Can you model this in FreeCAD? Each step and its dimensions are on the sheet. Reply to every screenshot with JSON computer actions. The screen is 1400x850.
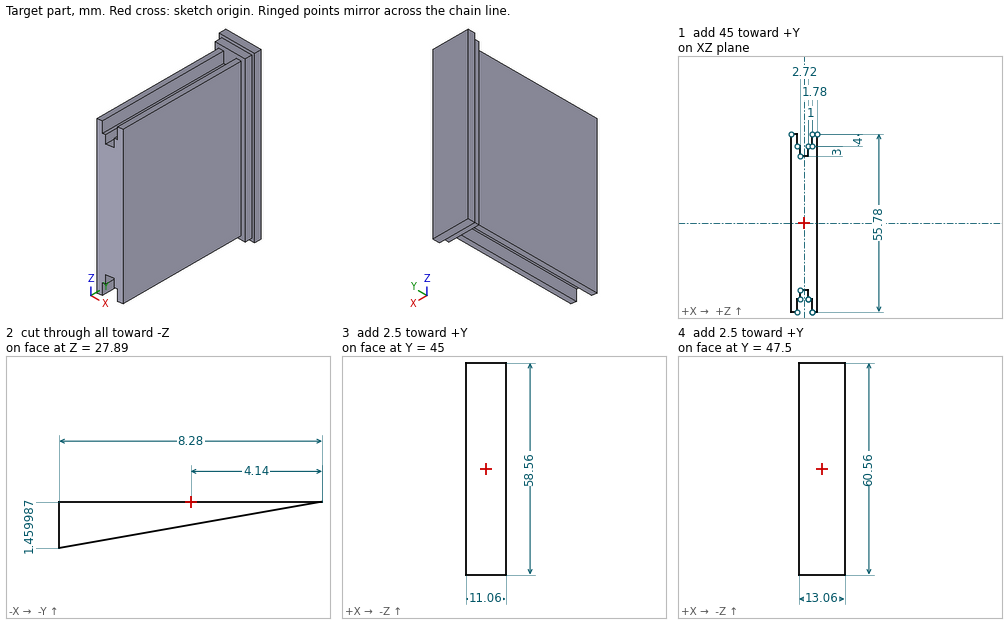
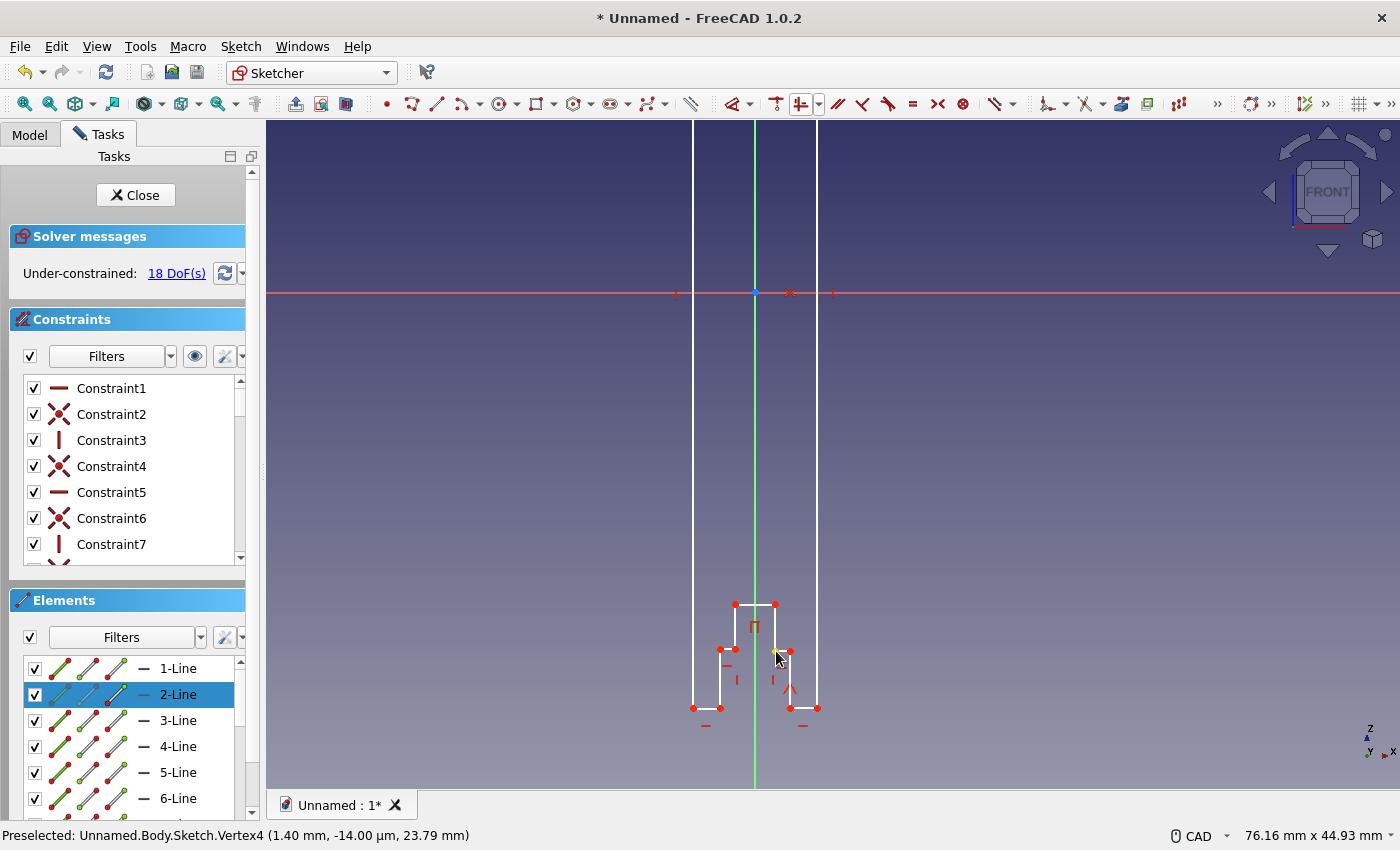
{"action": "left_click", "coordinate": [775, 651]}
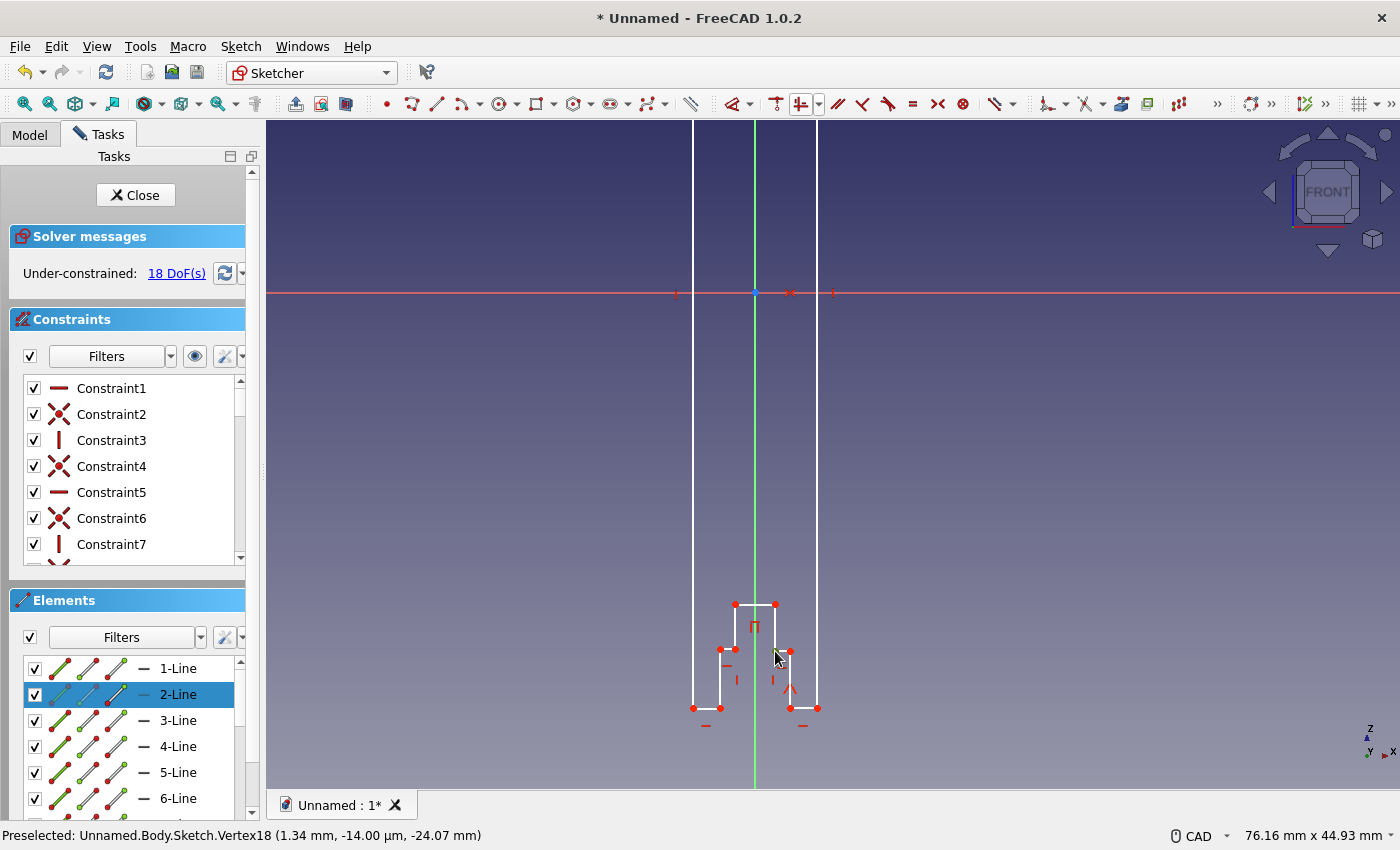
{"action": "left_click", "coordinate": [361, 293]}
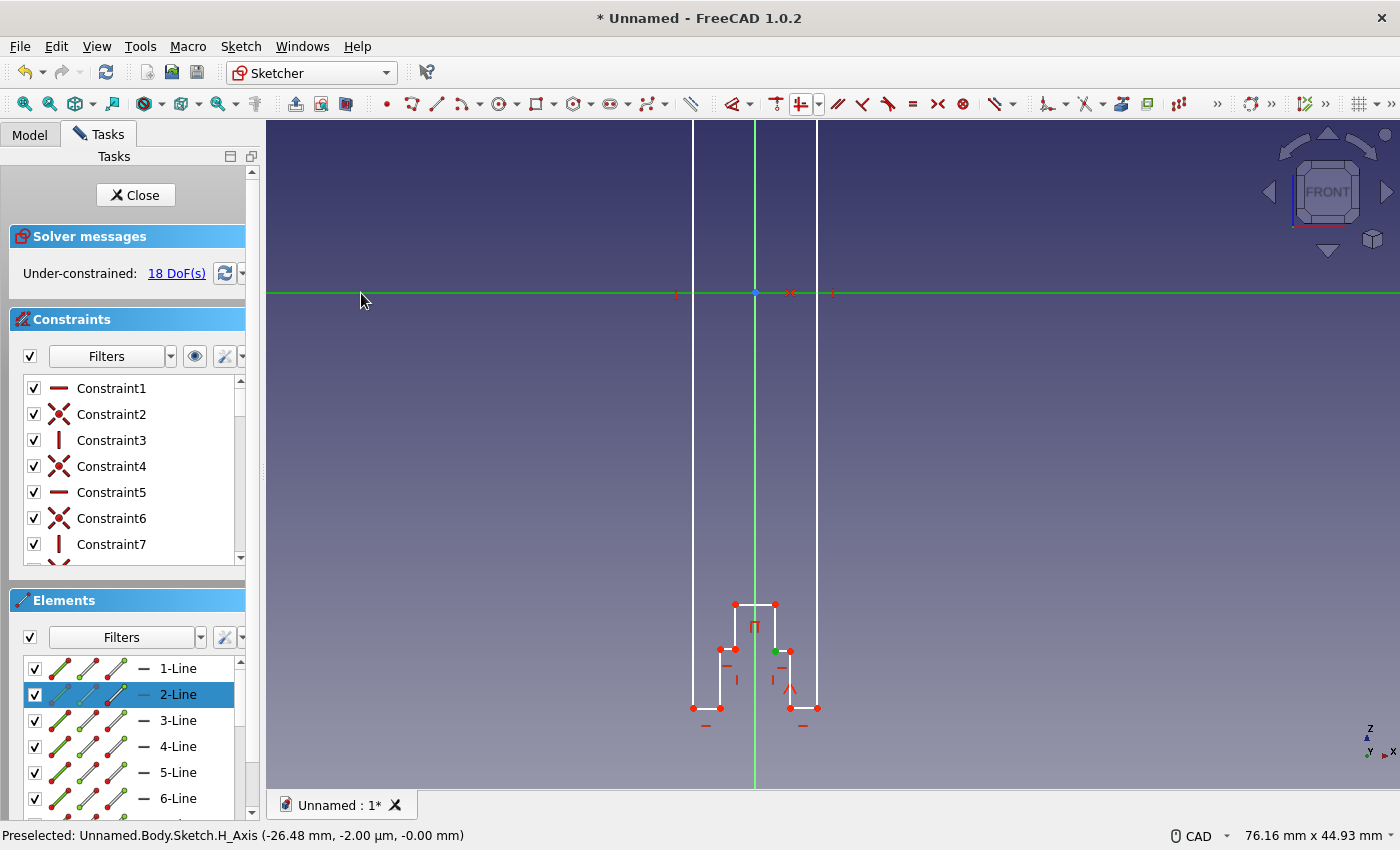
{"action": "left_click", "coordinate": [938, 104]}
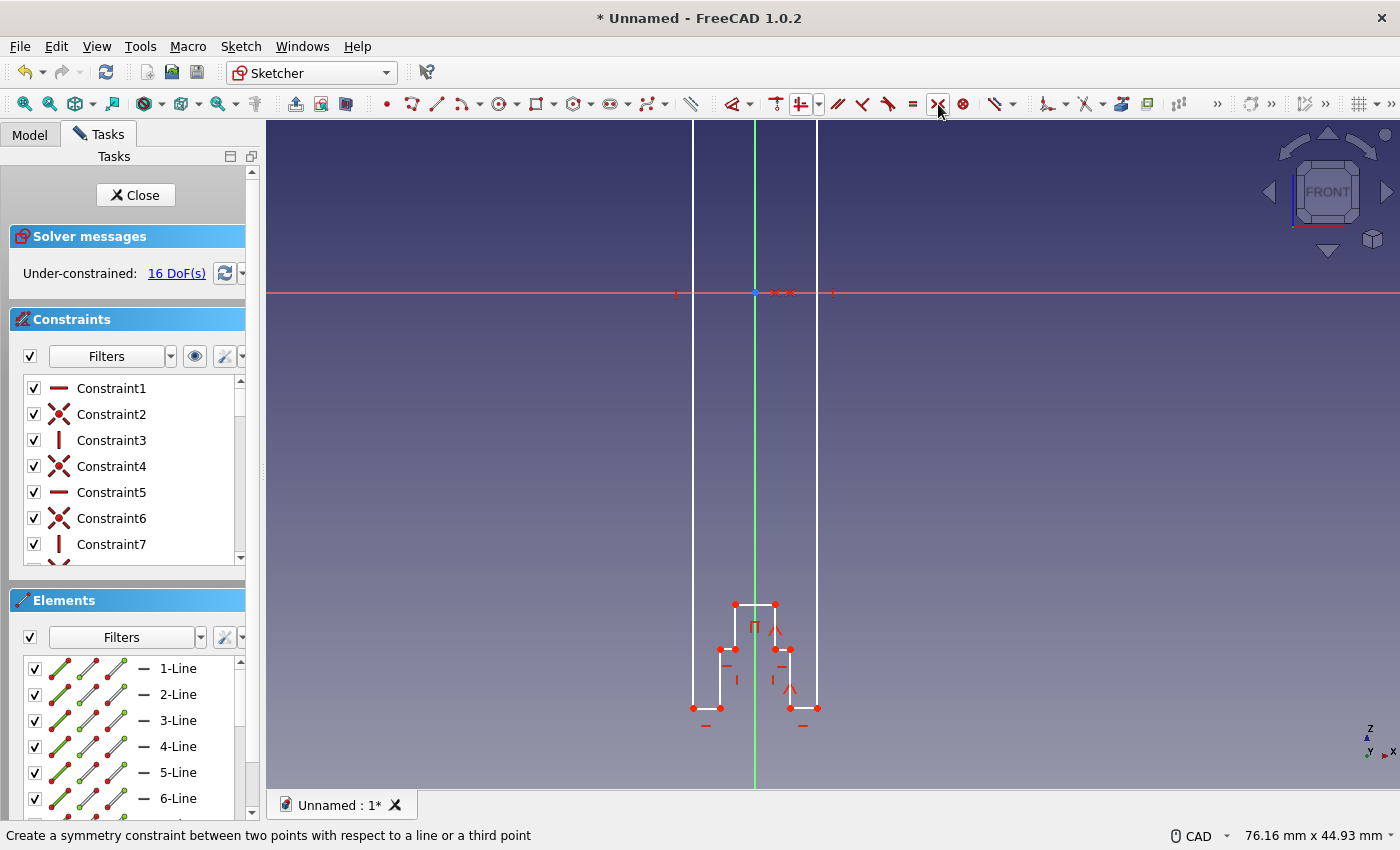
{"action": "scroll", "coordinate": [776, 651], "scroll_direction": "down", "scroll_amount": 3}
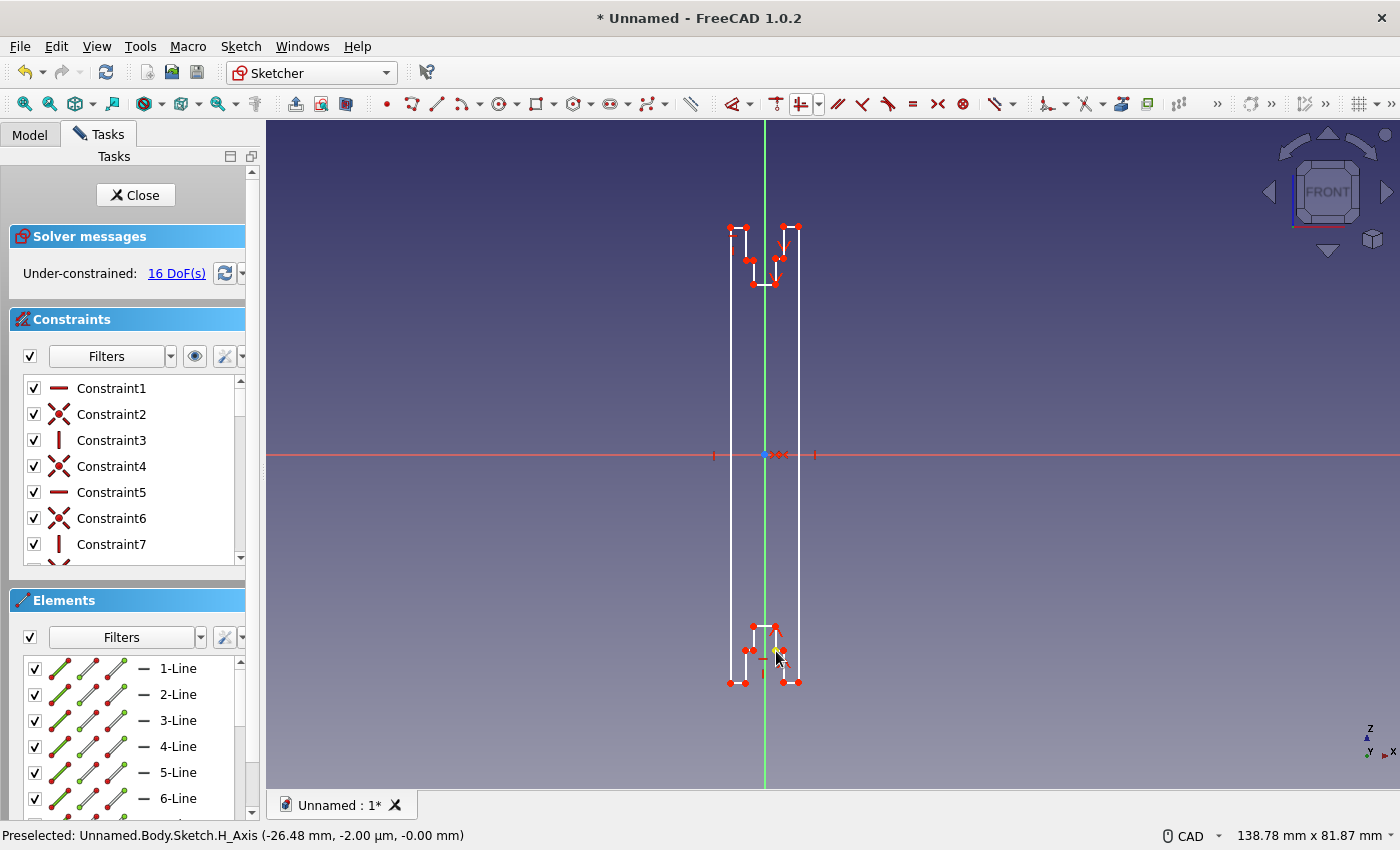
{"action": "left_click", "coordinate": [754, 284]}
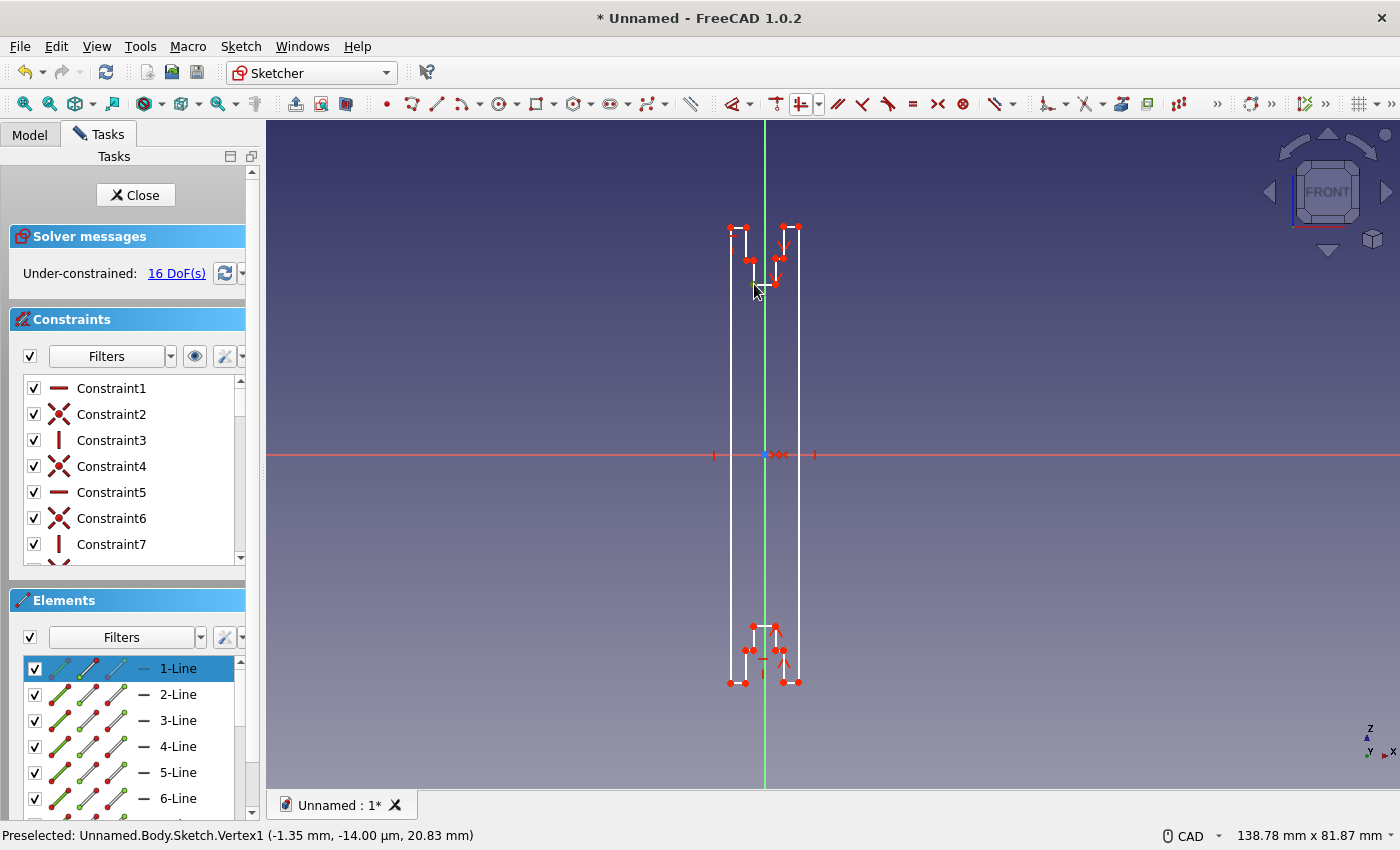
{"action": "left_click", "coordinate": [754, 626]}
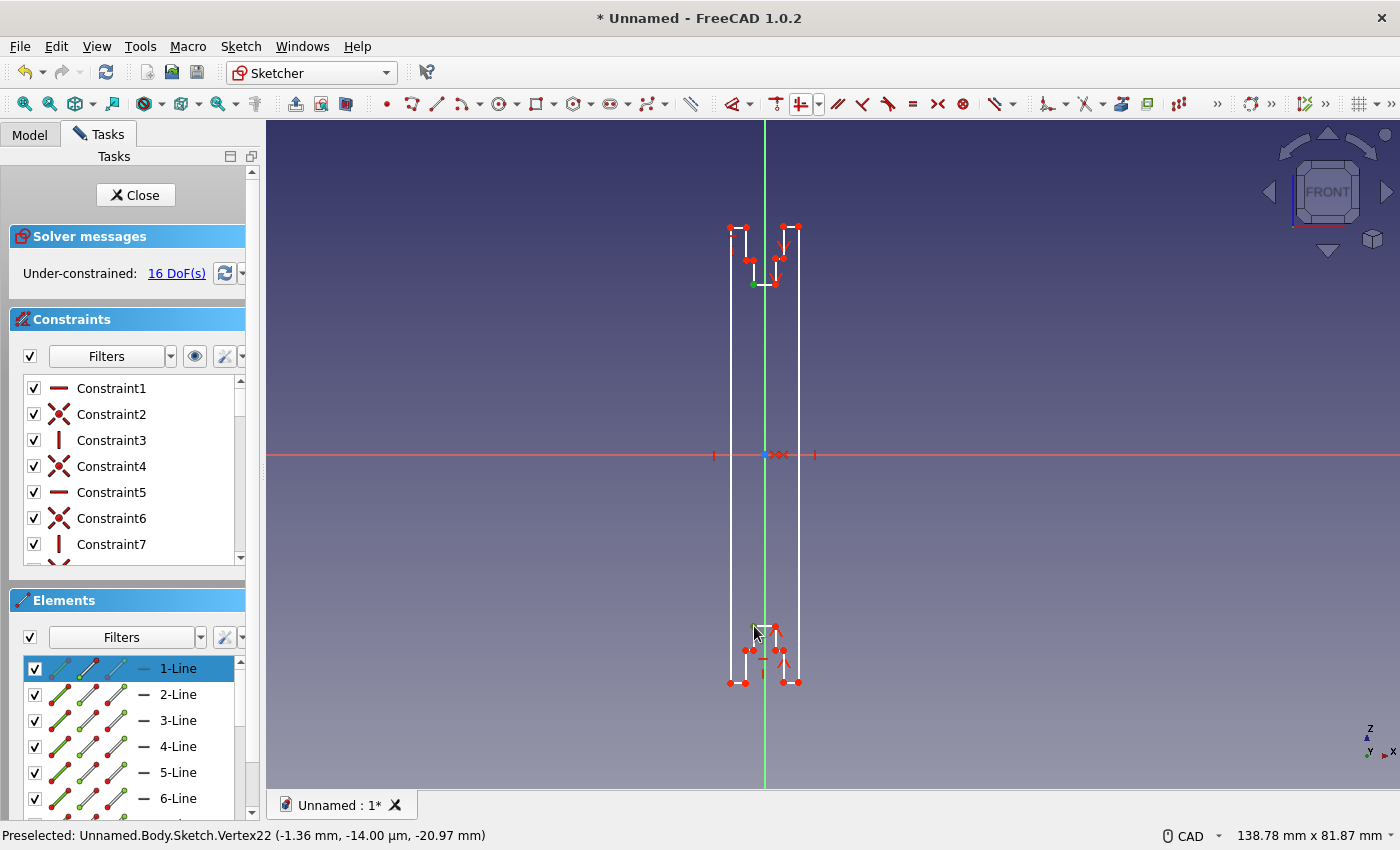
{"action": "left_click", "coordinate": [361, 455]}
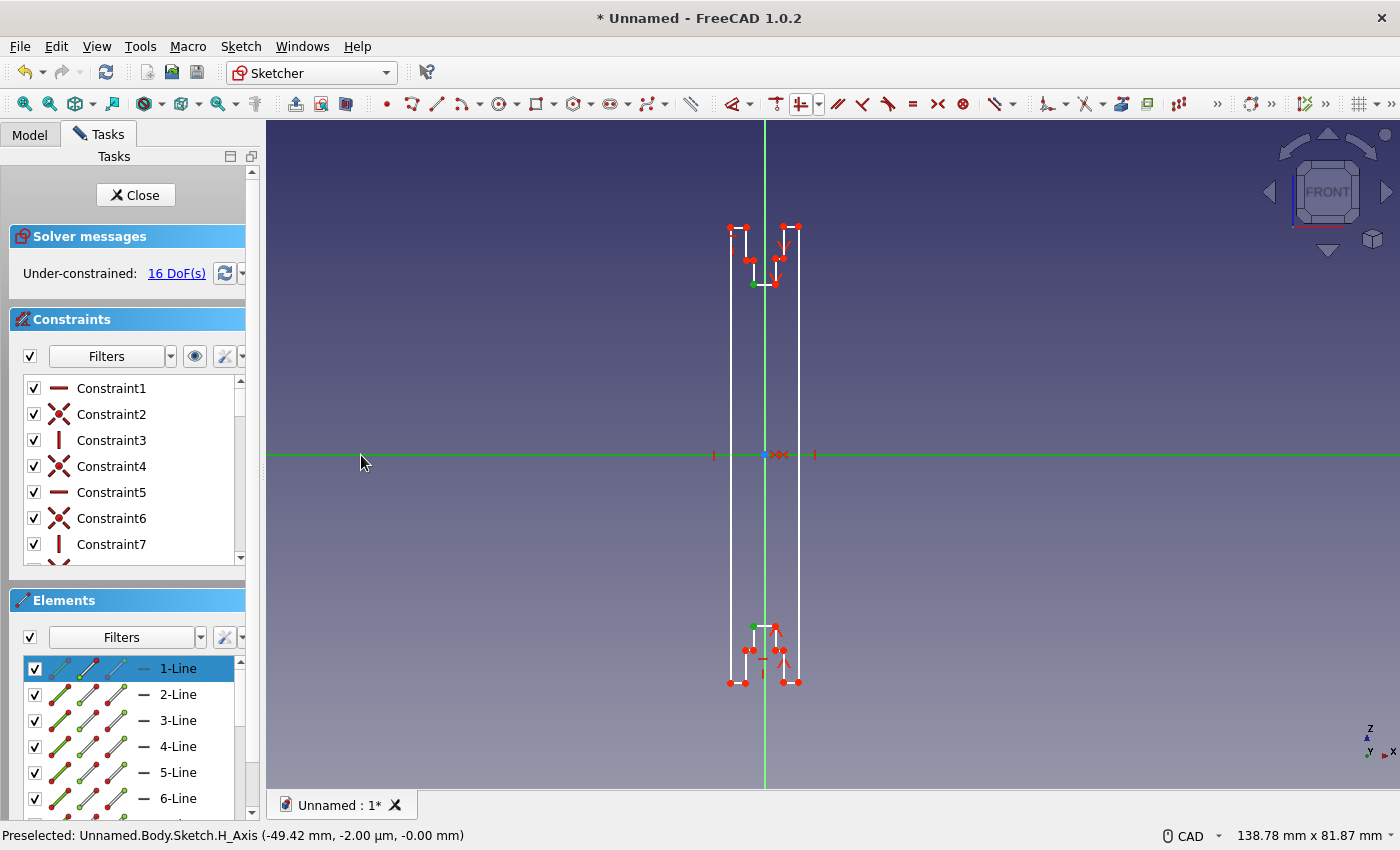
{"action": "key", "text": "s"}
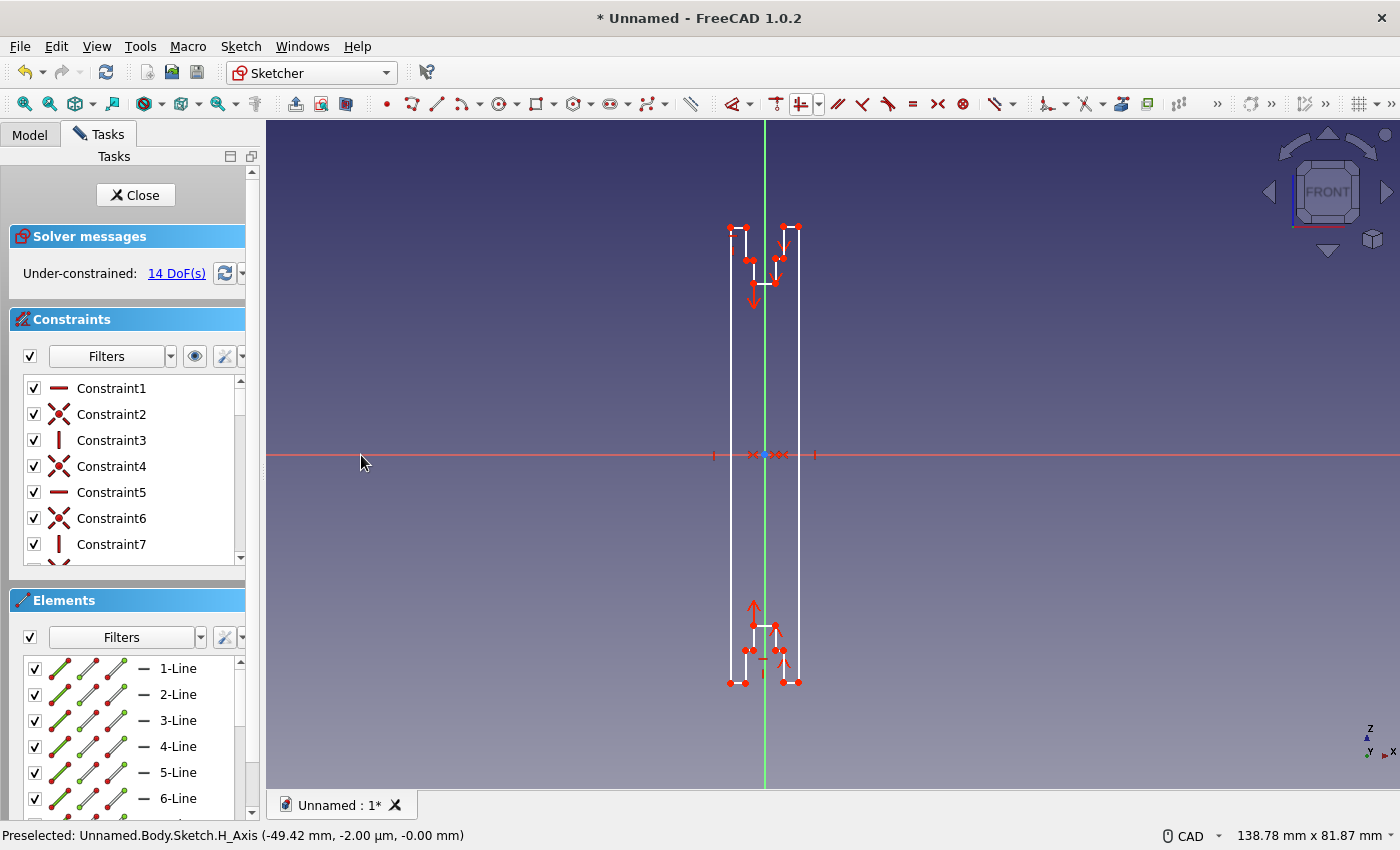
{"action": "scroll", "coordinate": [776, 651], "scroll_direction": "up", "scroll_amount": 3}